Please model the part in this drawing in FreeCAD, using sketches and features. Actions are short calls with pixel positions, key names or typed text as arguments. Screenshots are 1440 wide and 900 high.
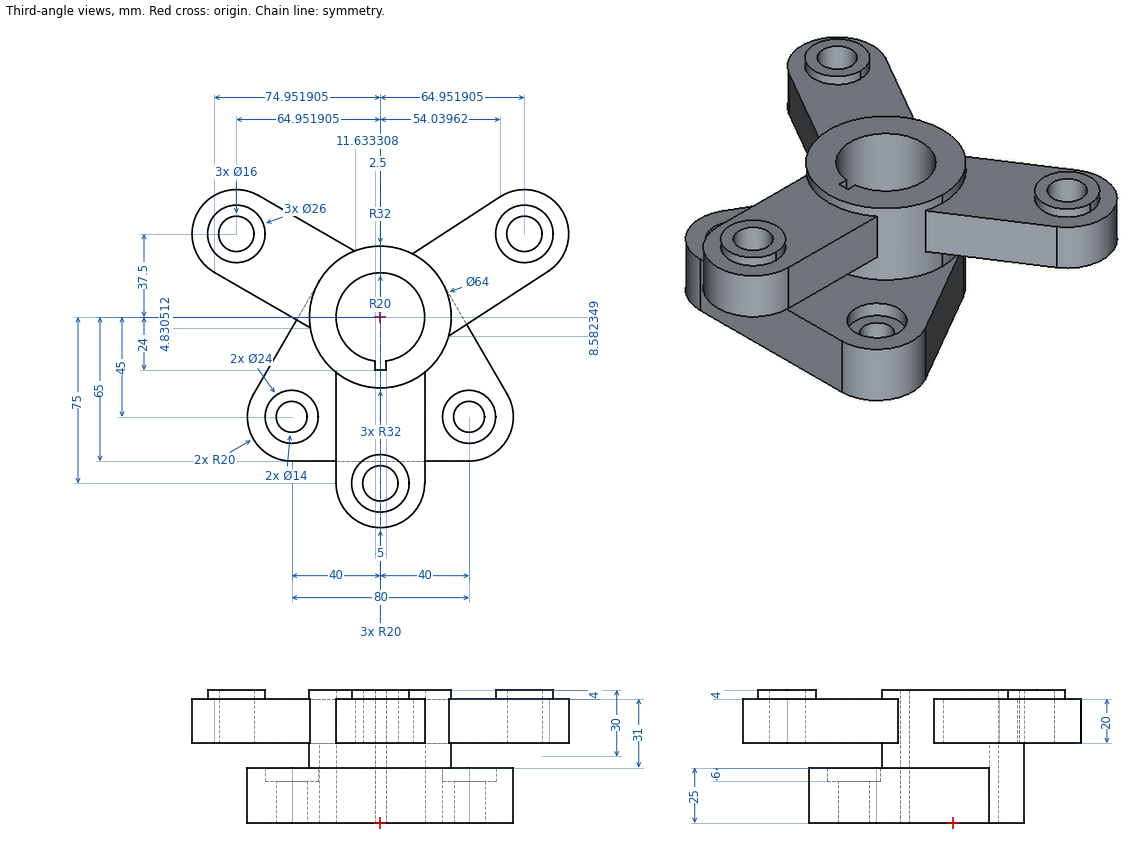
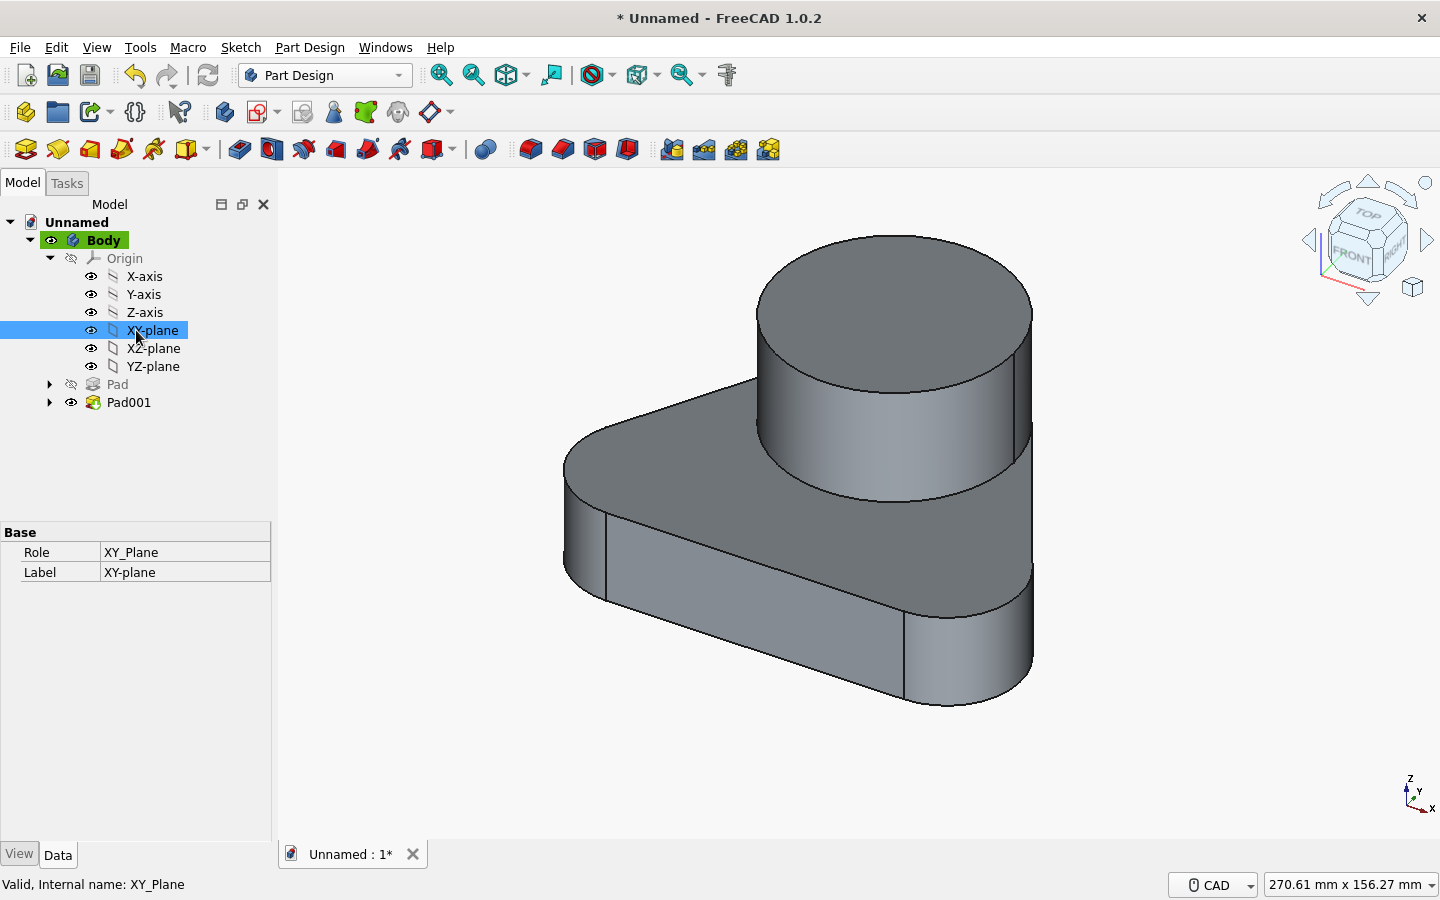
click(430, 112)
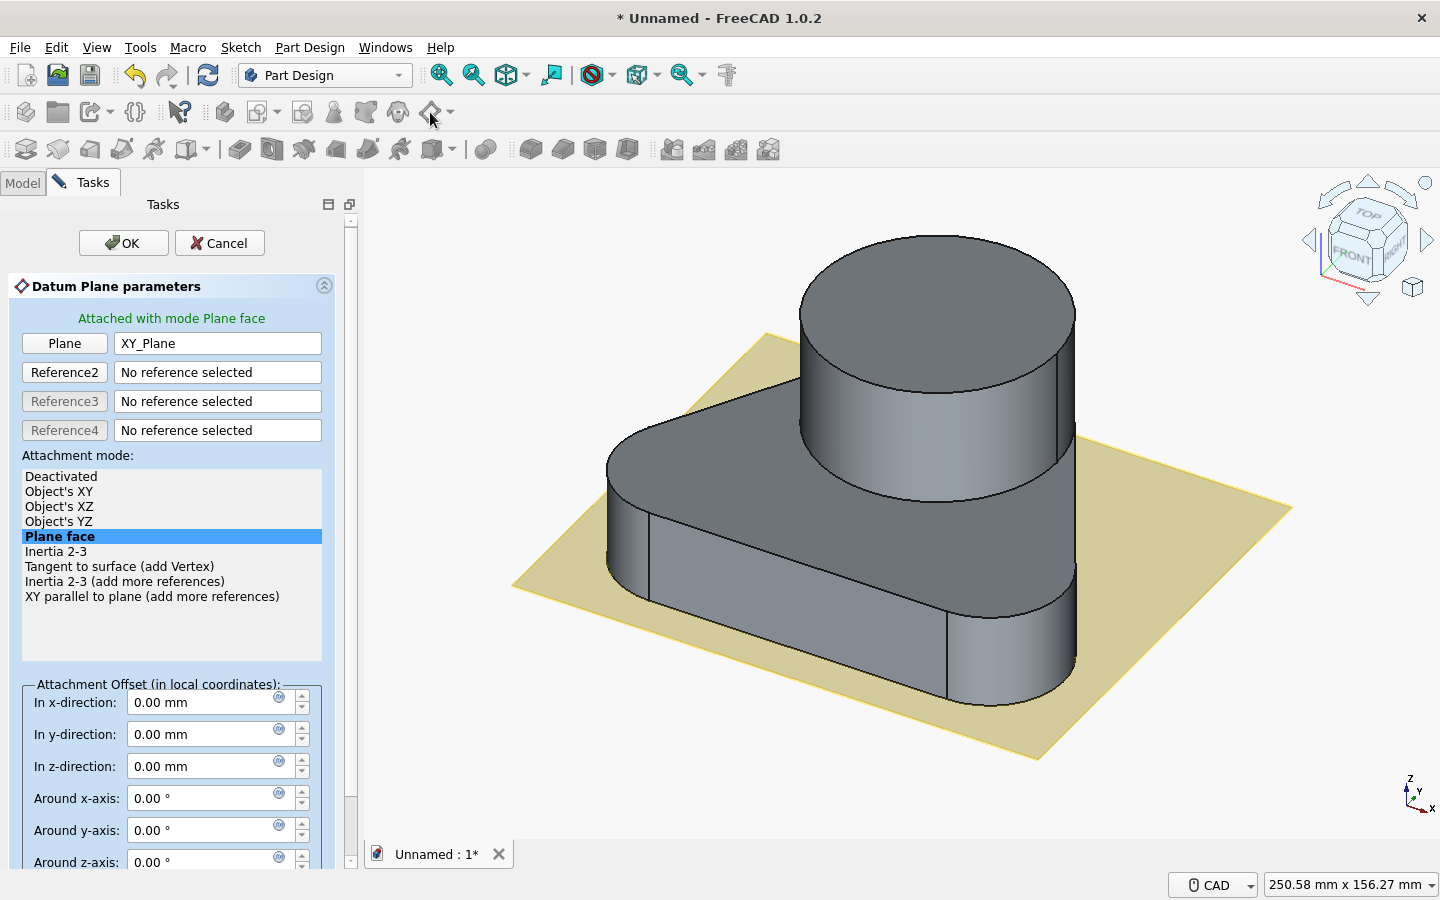
triple_click(210, 766)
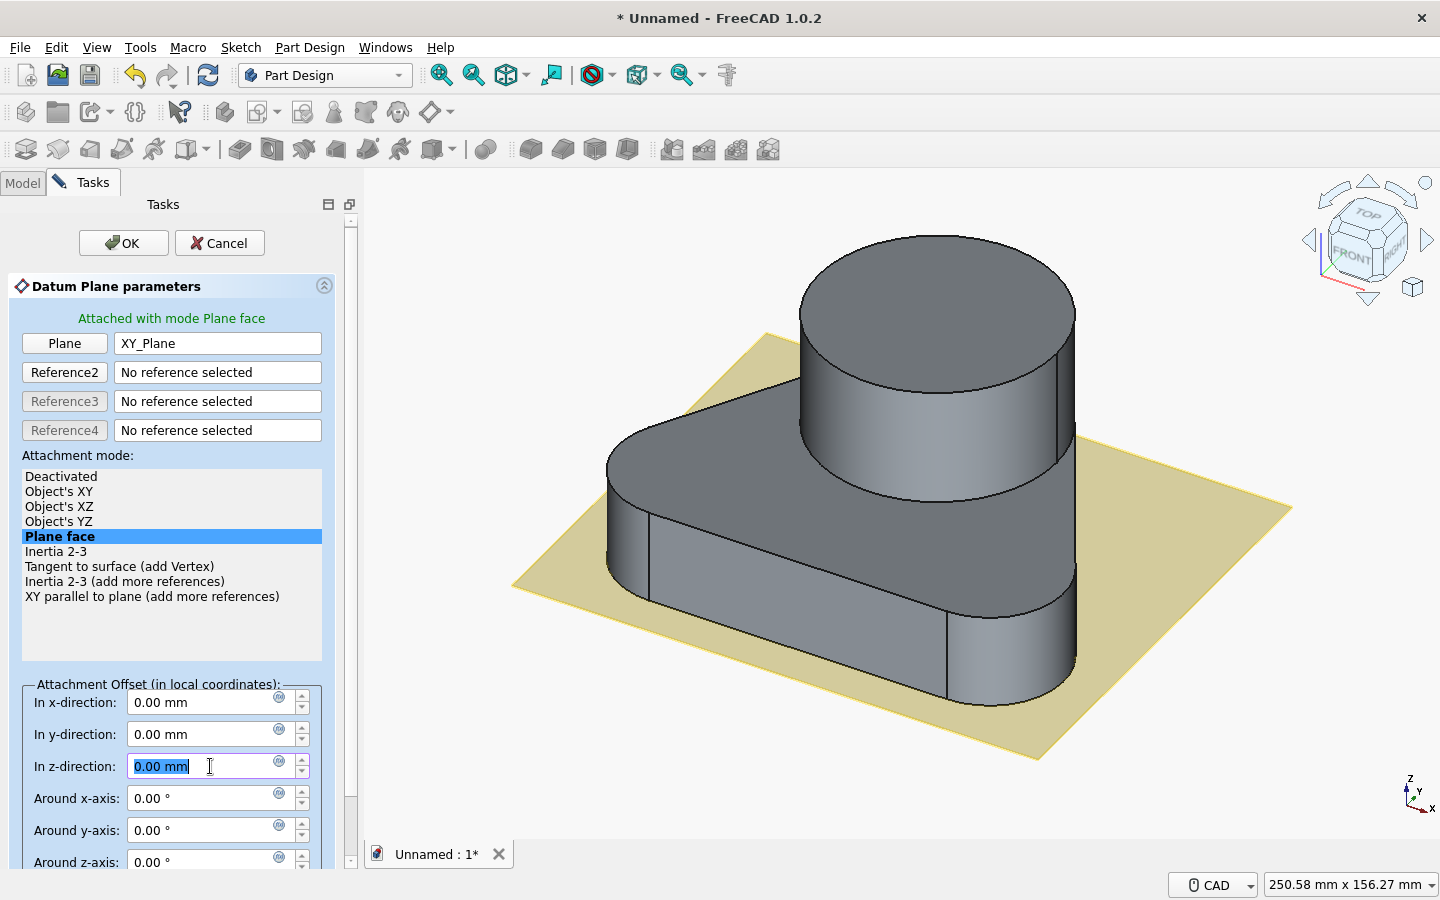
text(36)
key(Tab)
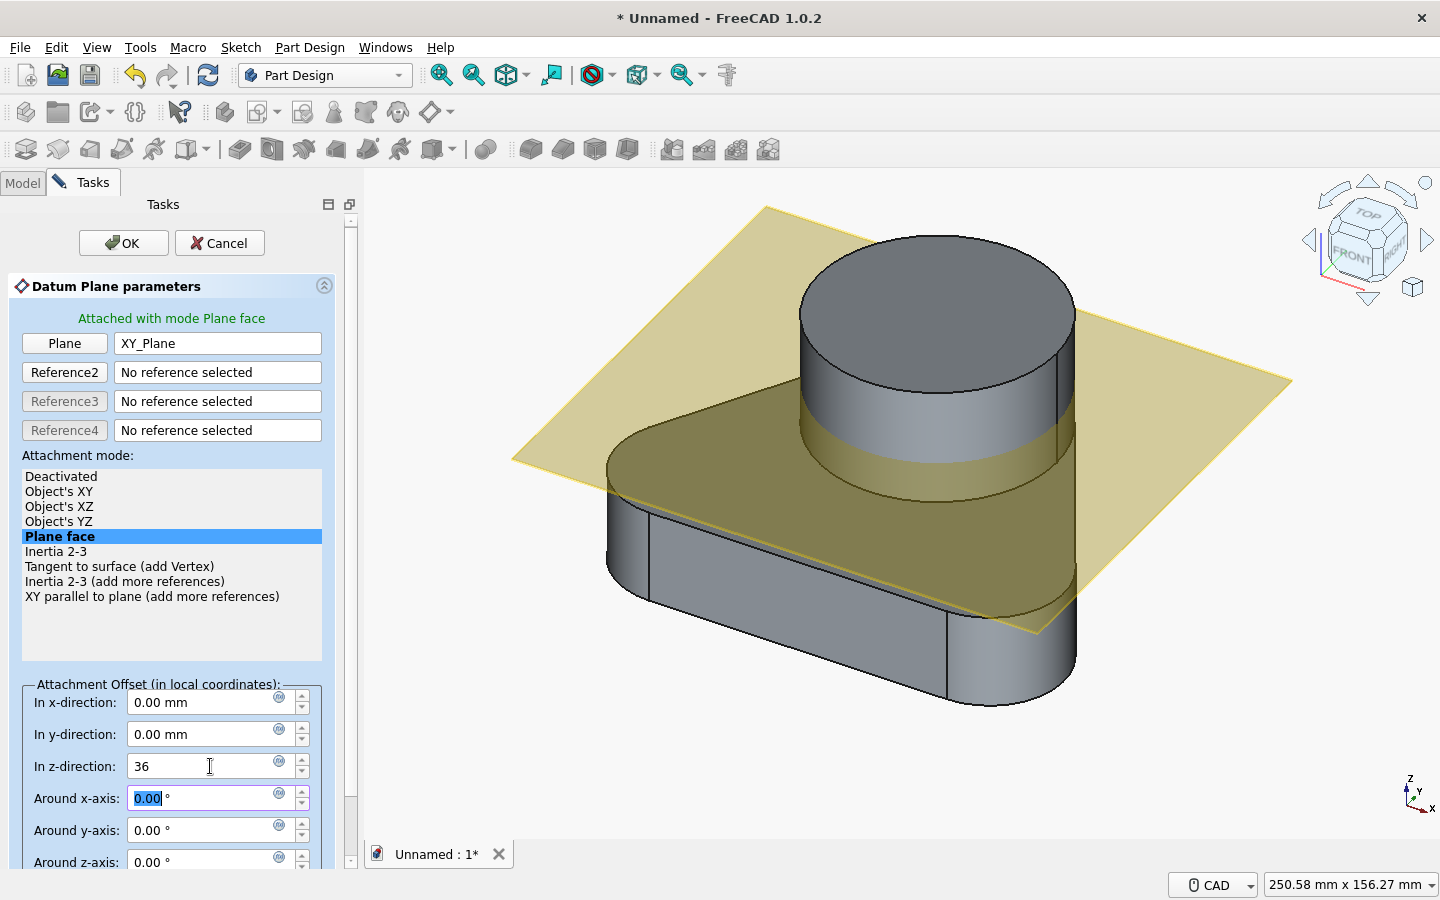
click(124, 243)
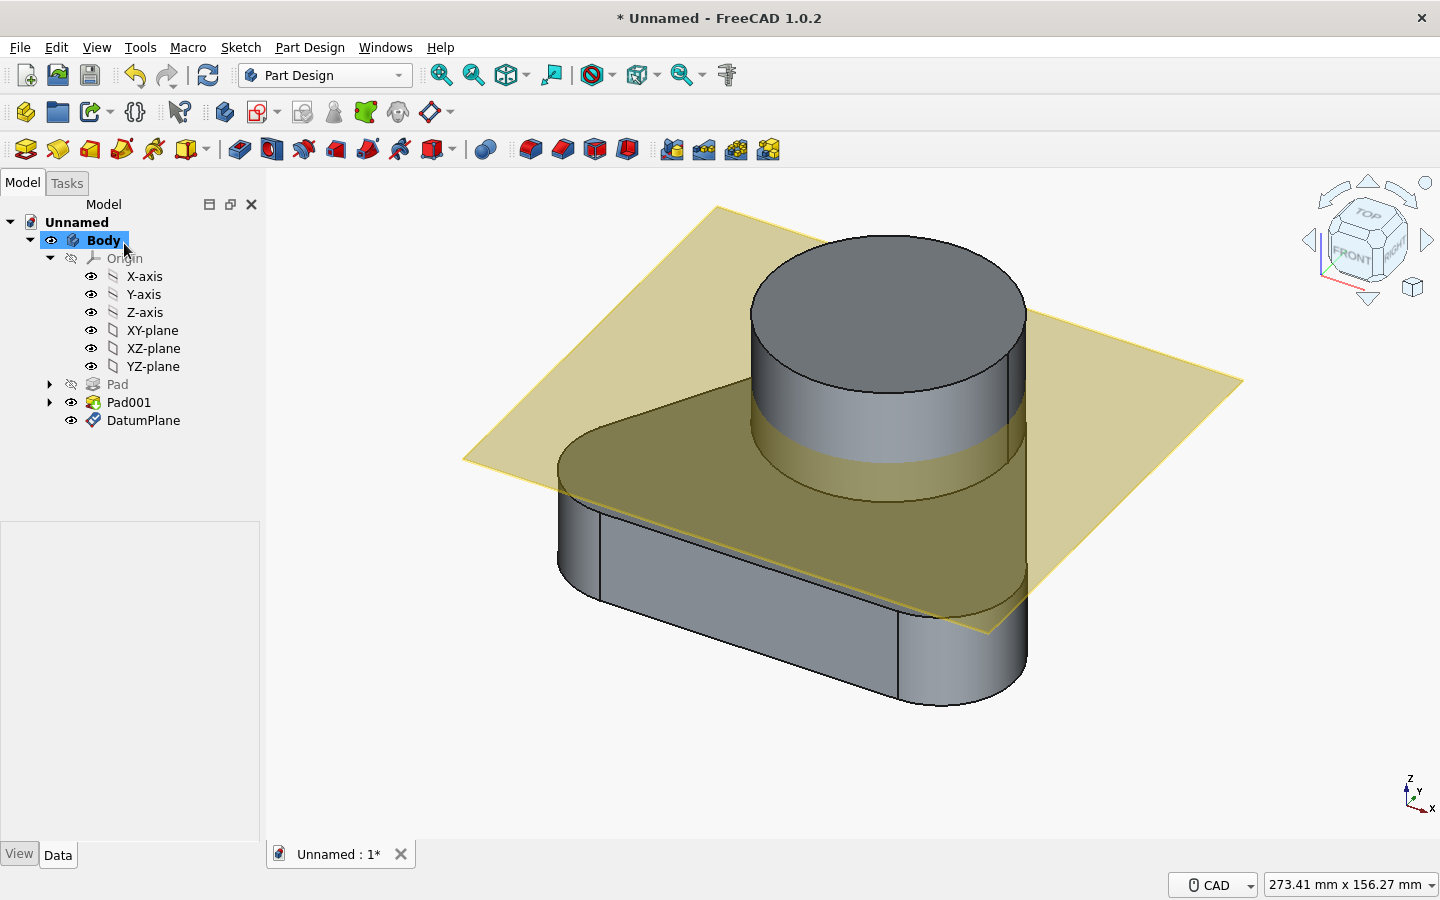
click(116, 420)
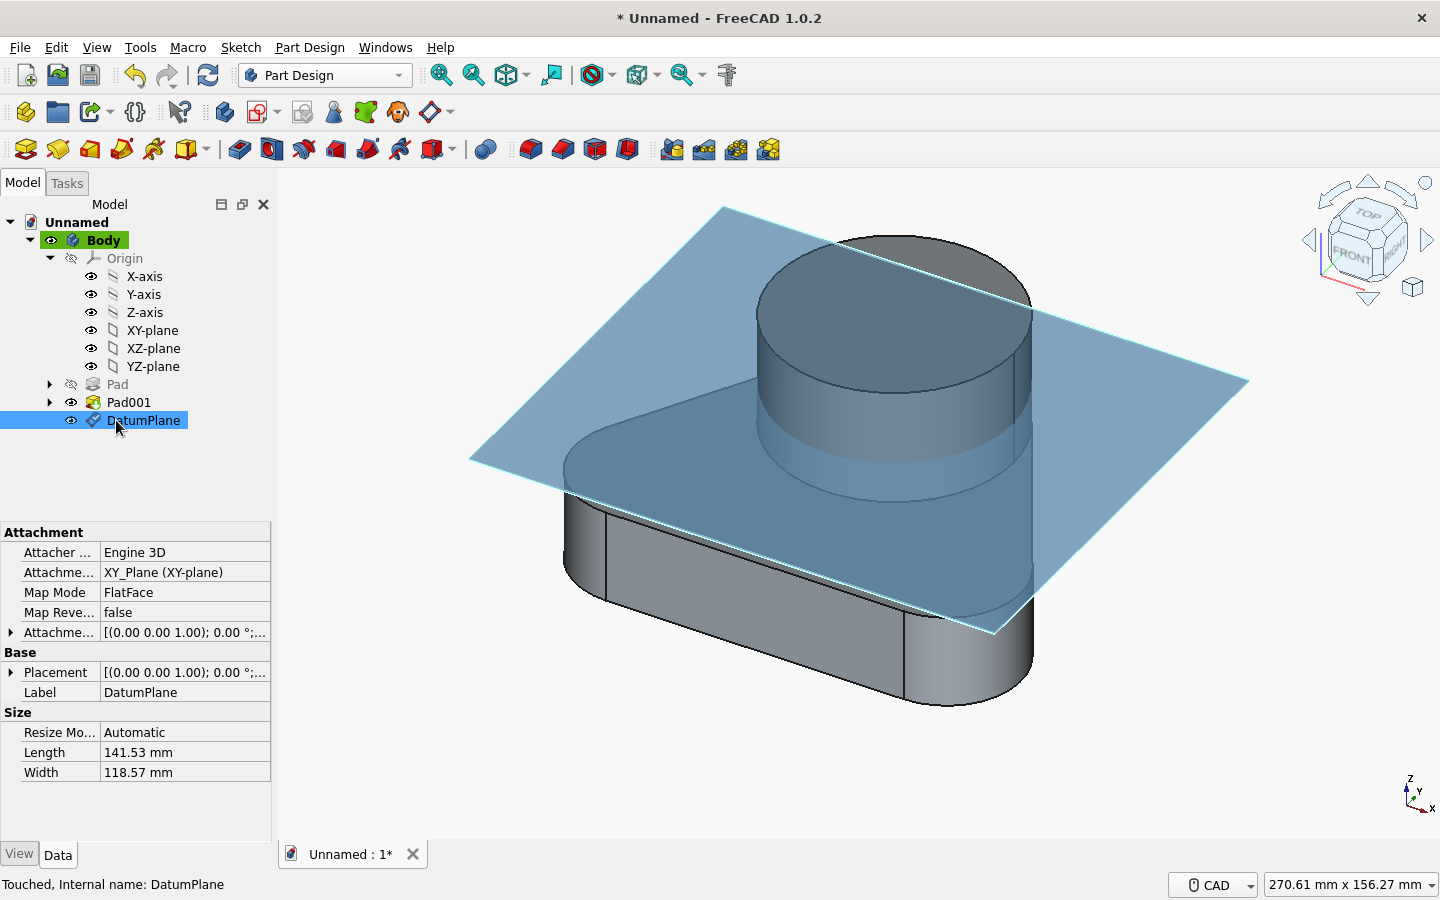
click(258, 112)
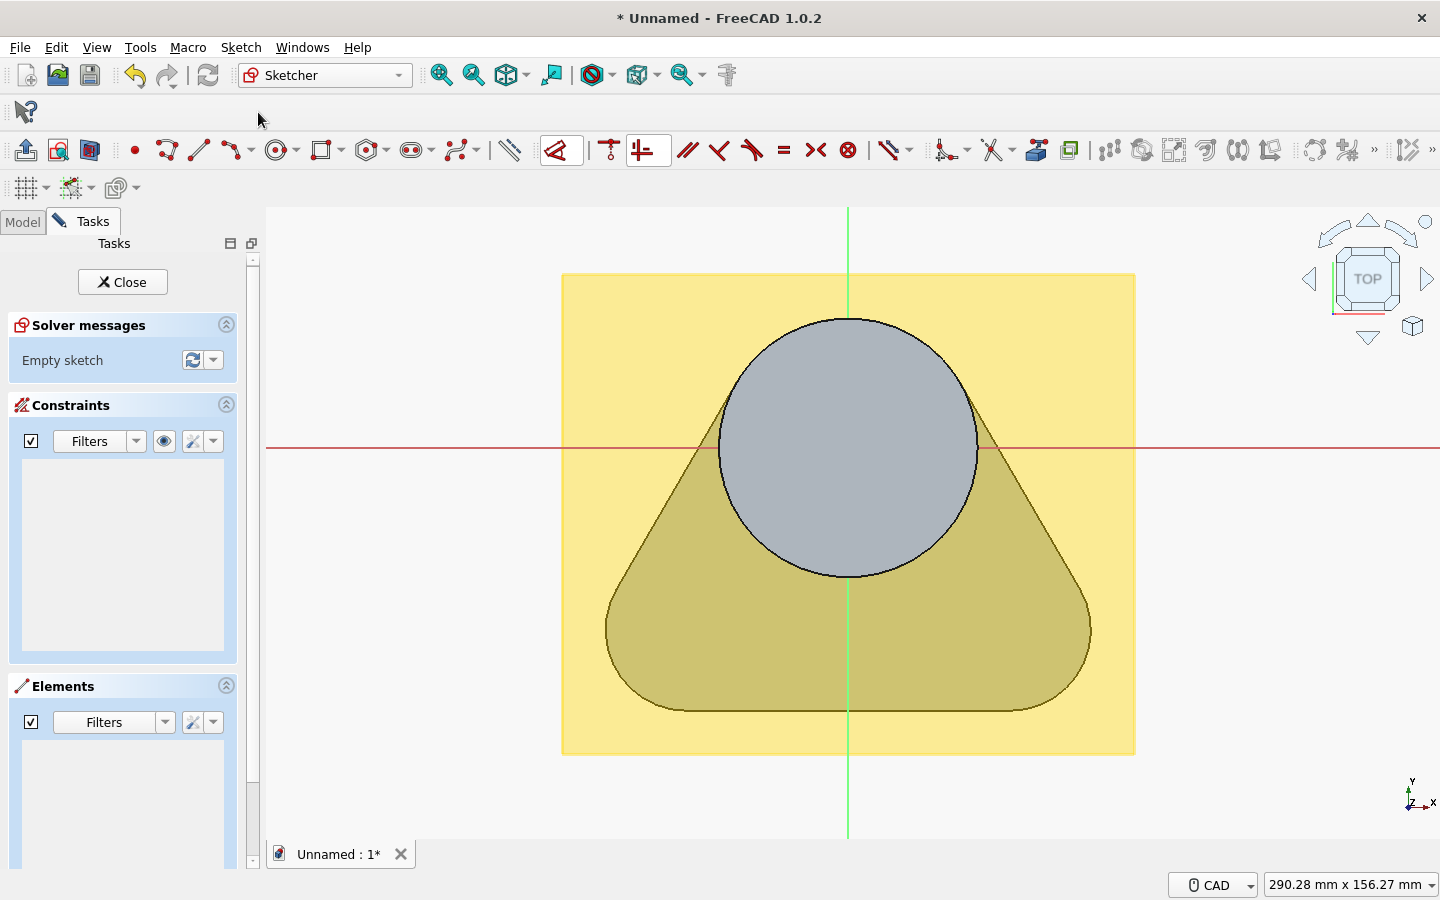
click(90, 150)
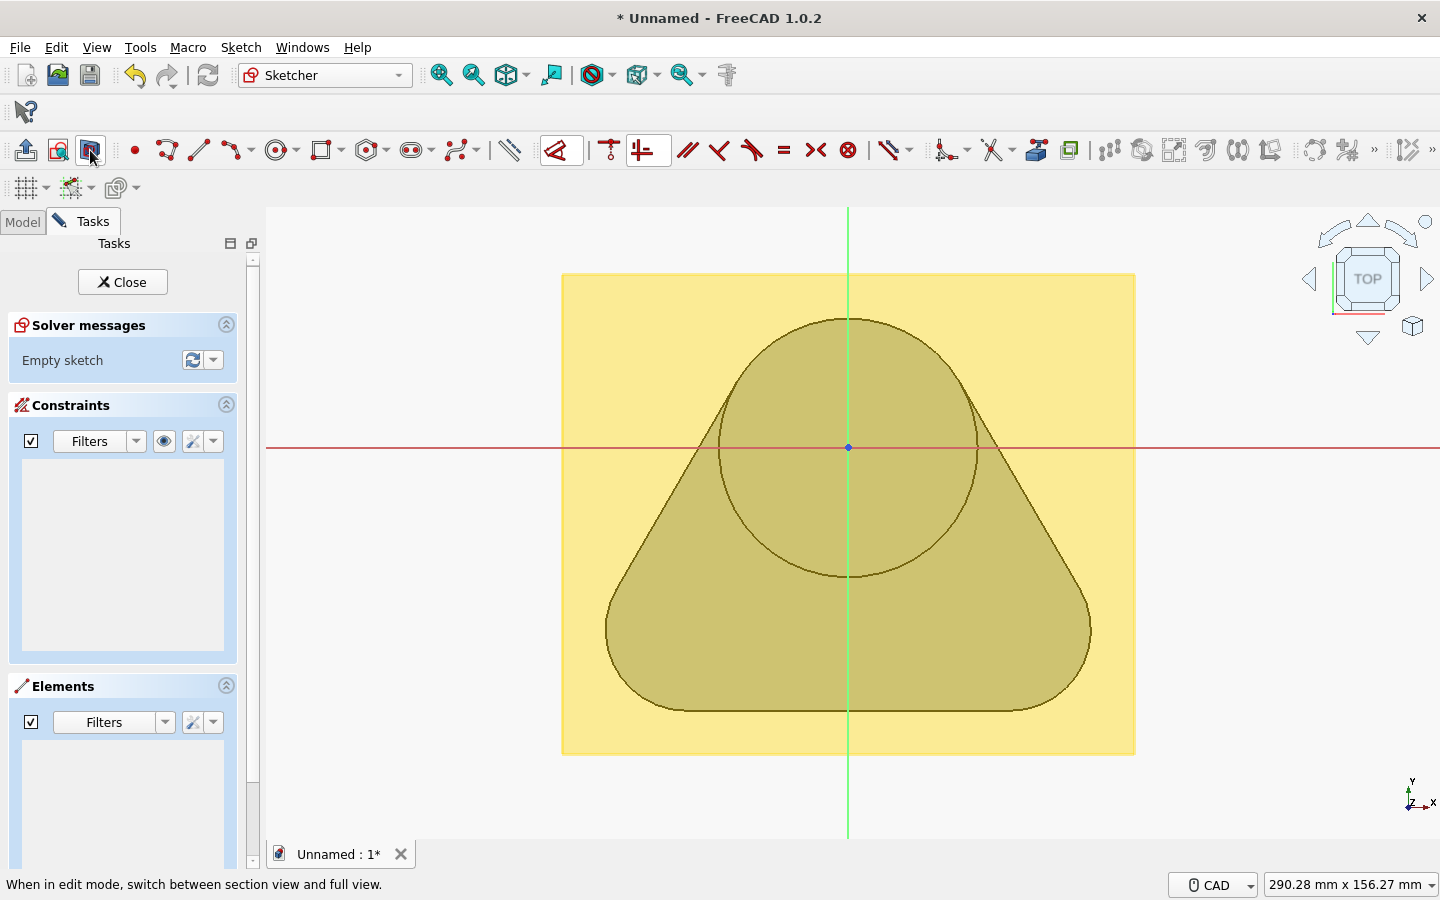
scroll(657, 511, down, 2)